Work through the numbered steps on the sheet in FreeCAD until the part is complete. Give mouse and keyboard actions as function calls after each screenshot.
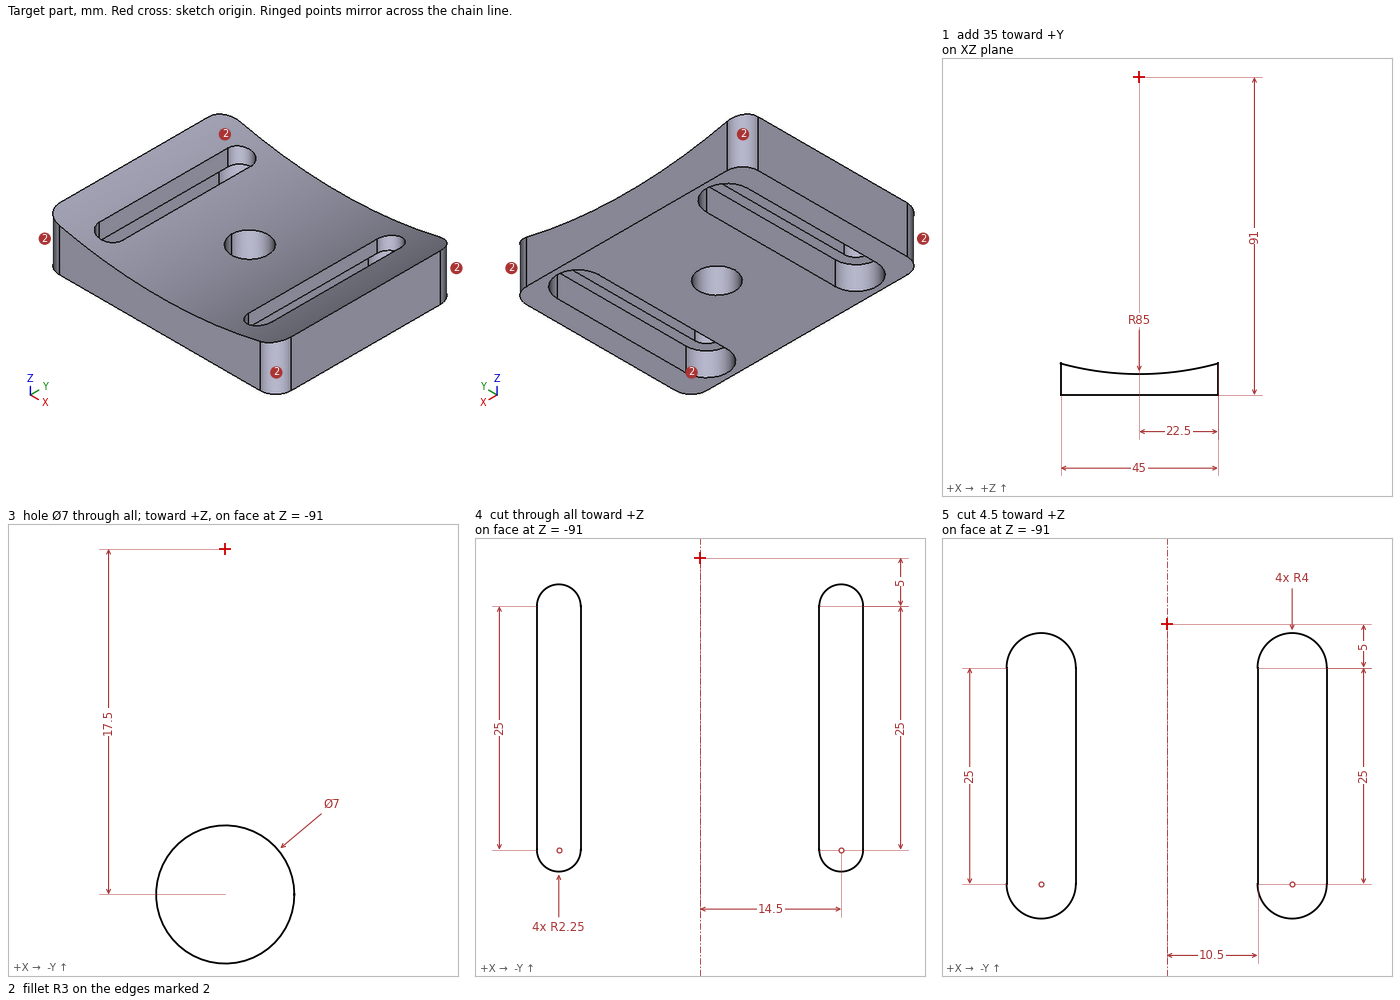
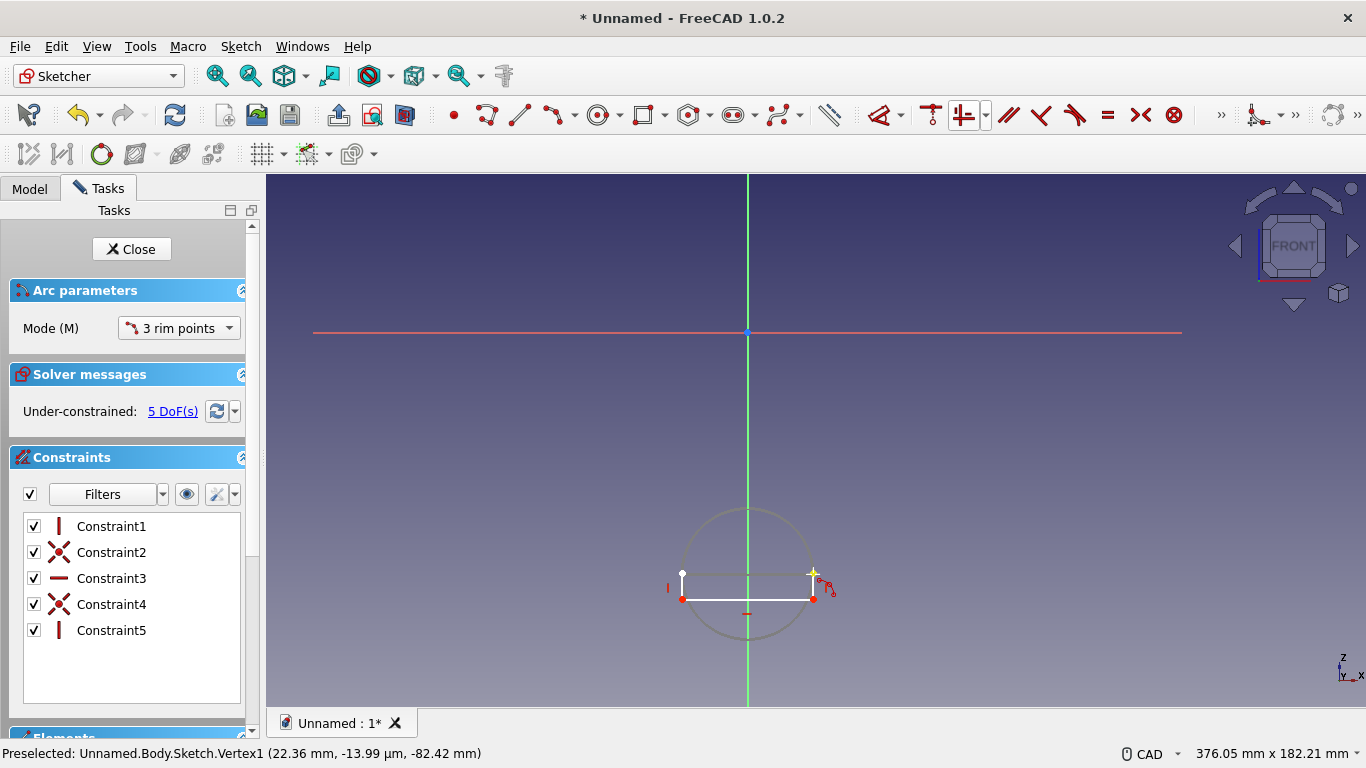
scroll(734, 581, up, 4)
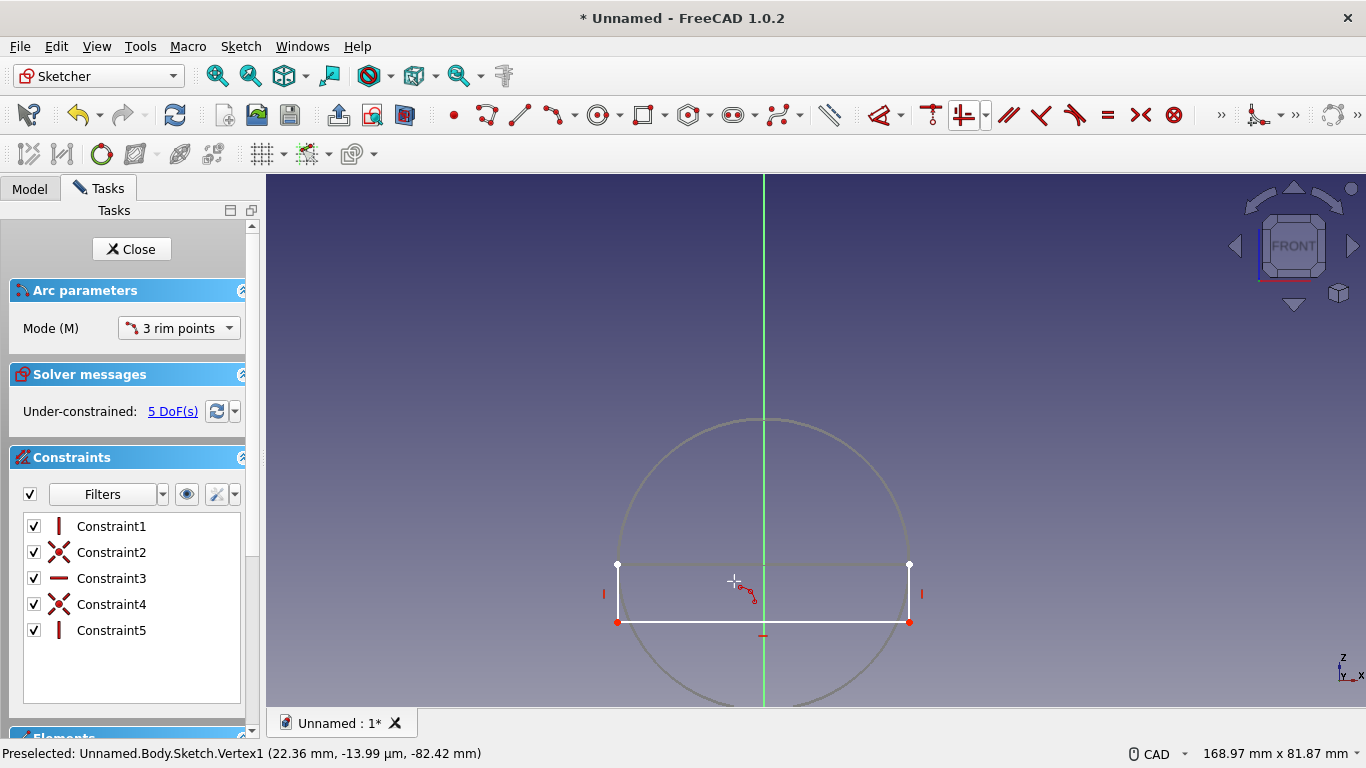
click(734, 581)
key(Escape)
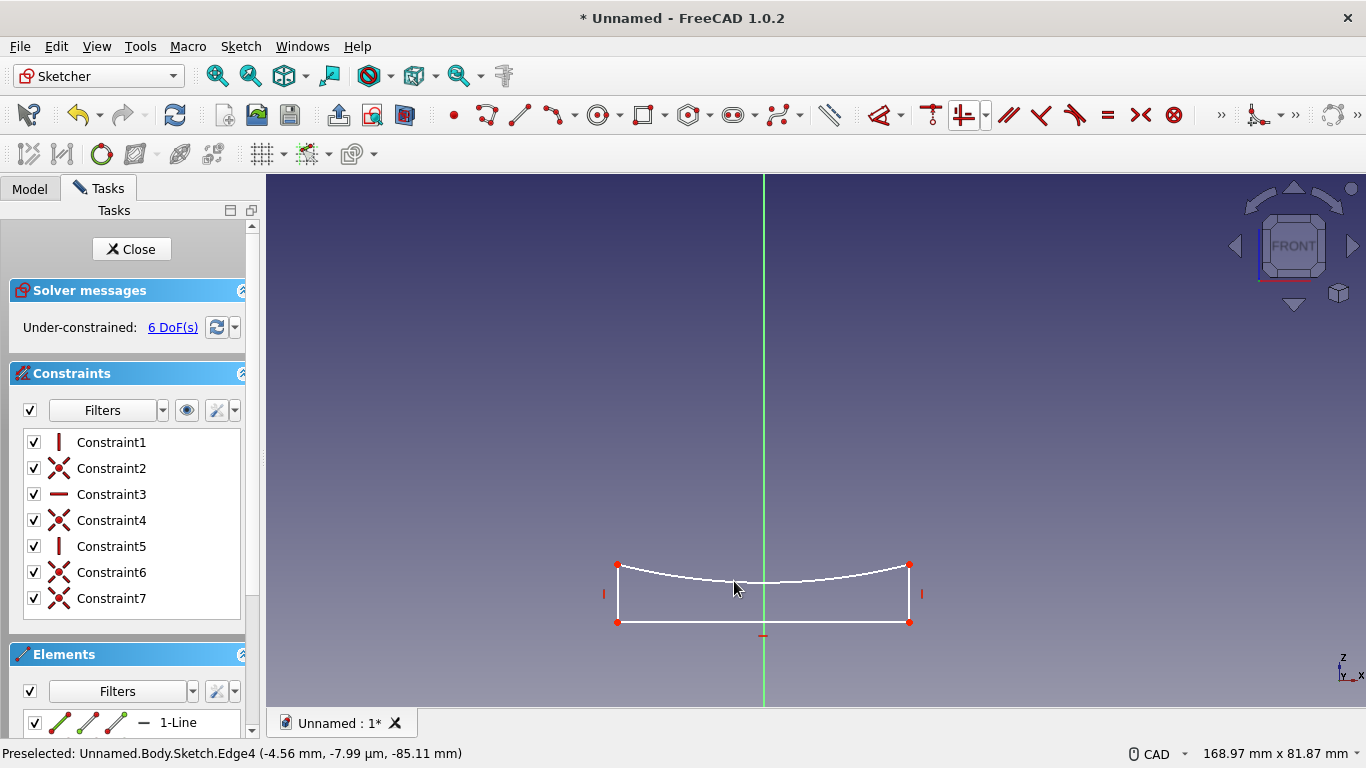
scroll(728, 582, down, 3)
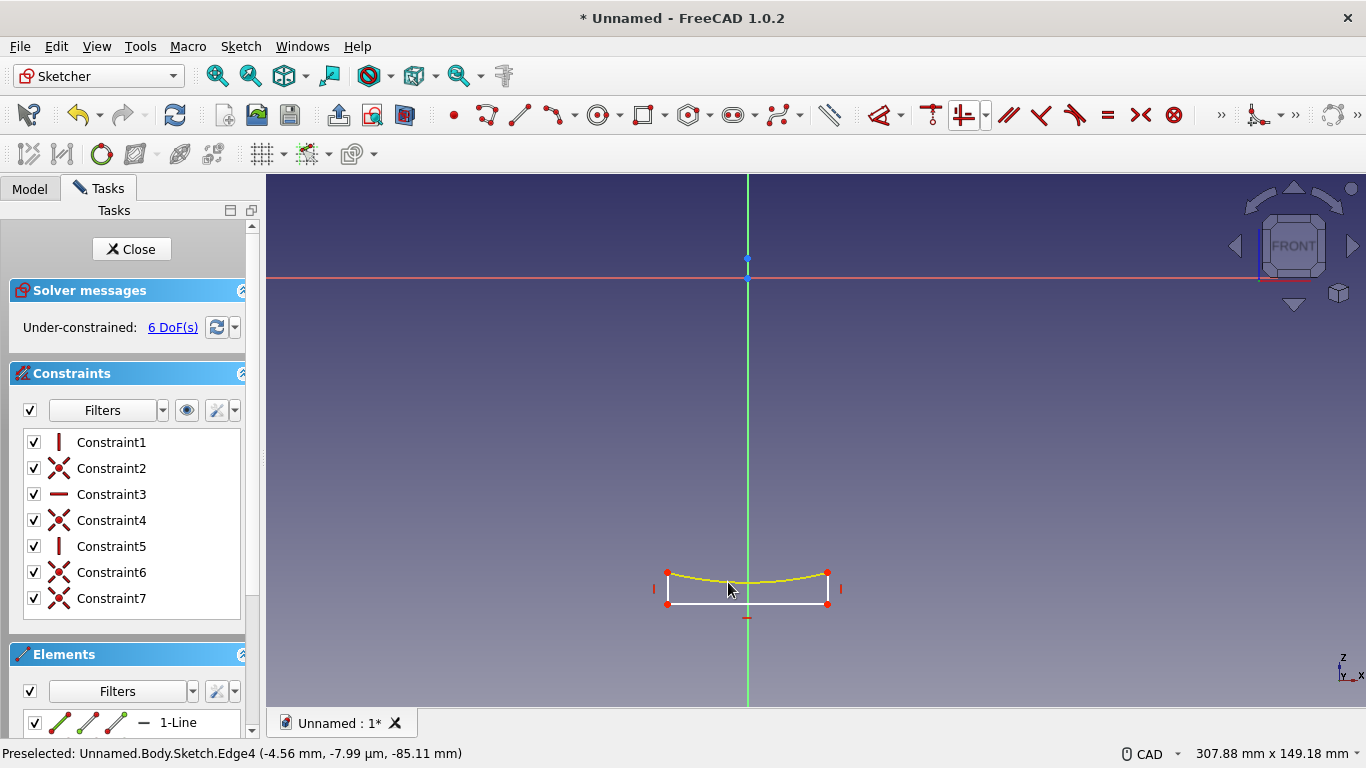
drag(738, 248, 758, 288)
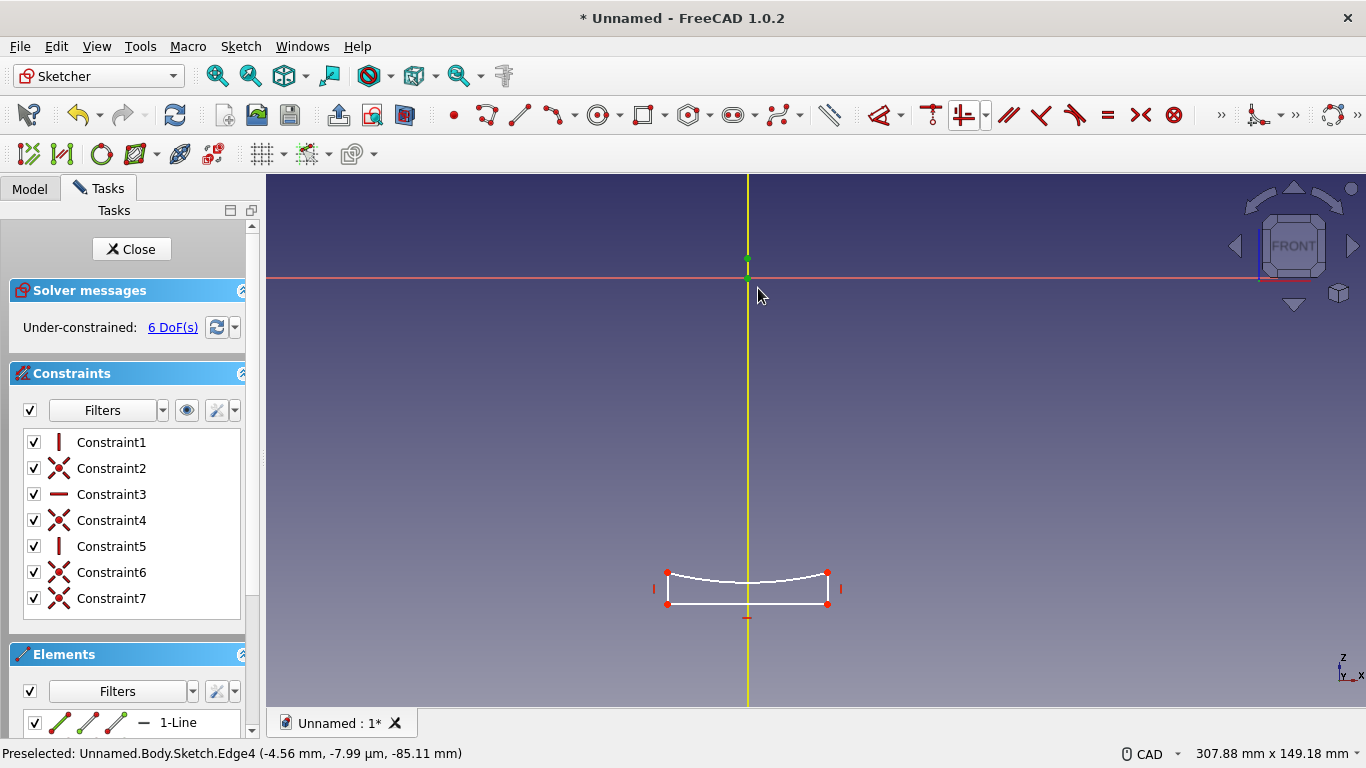
key(c)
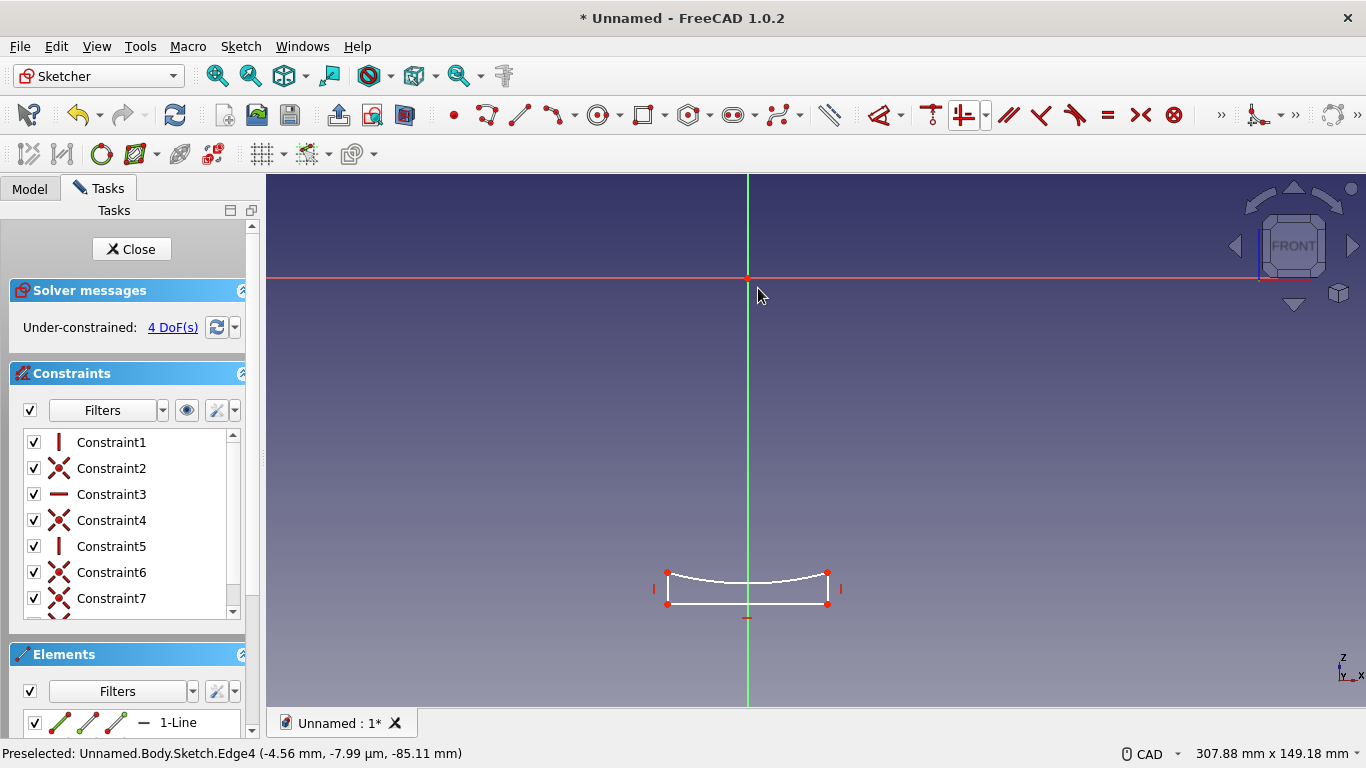
click(878, 116)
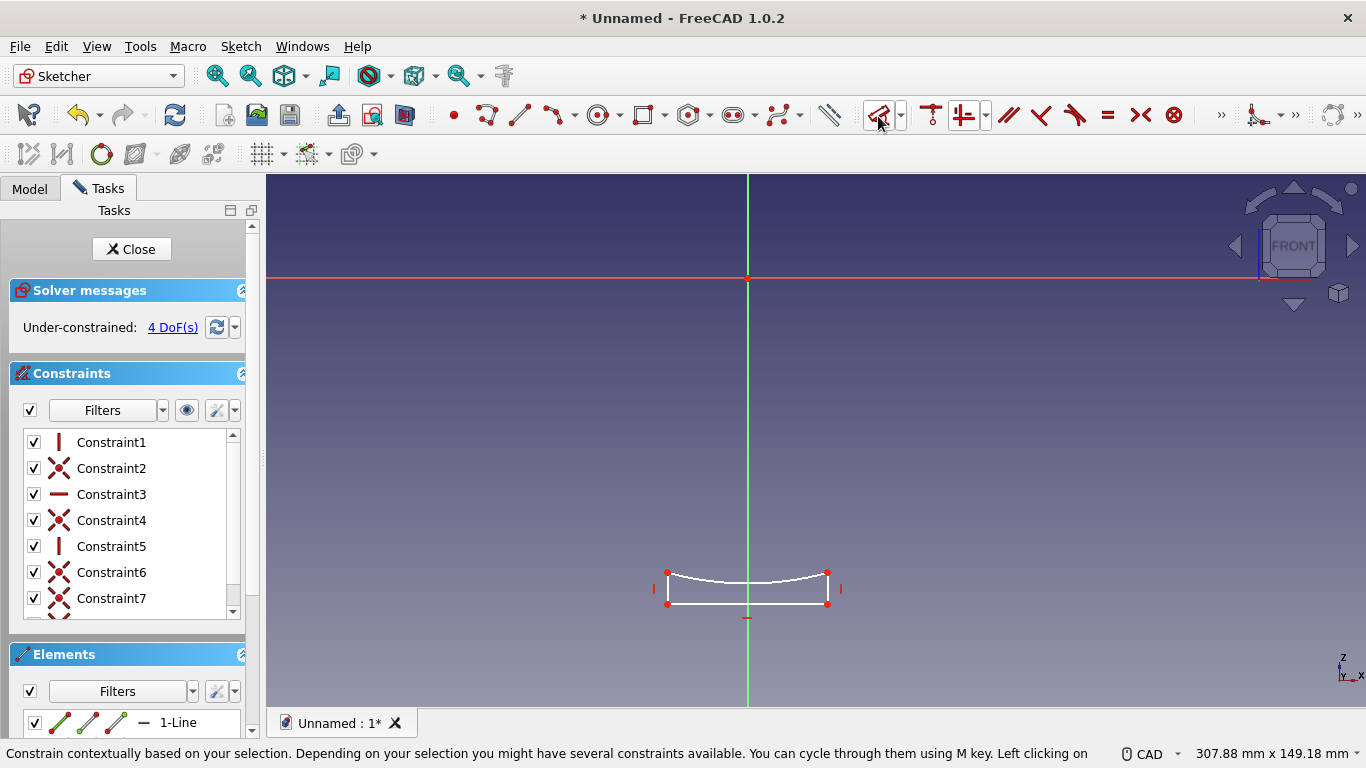
click(715, 582)
click(555, 555)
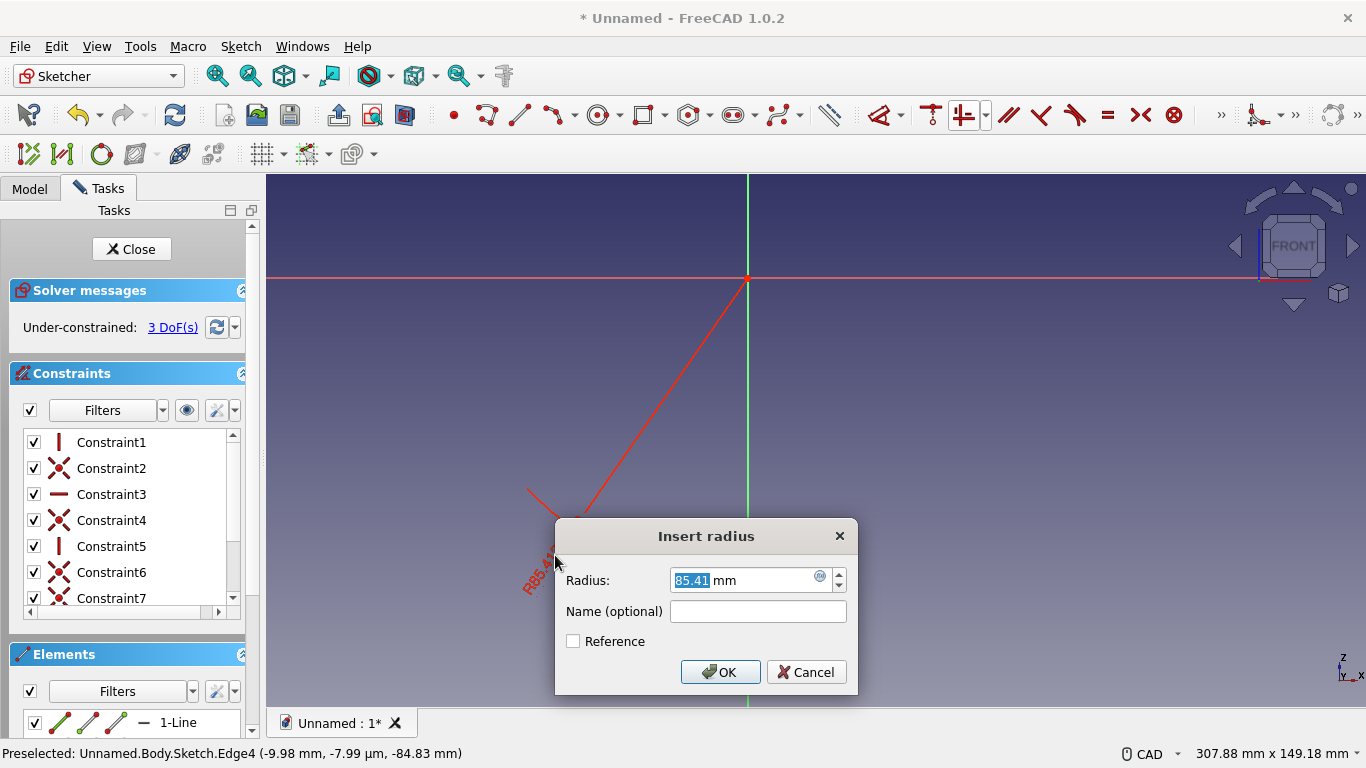
text(85)
key(Return)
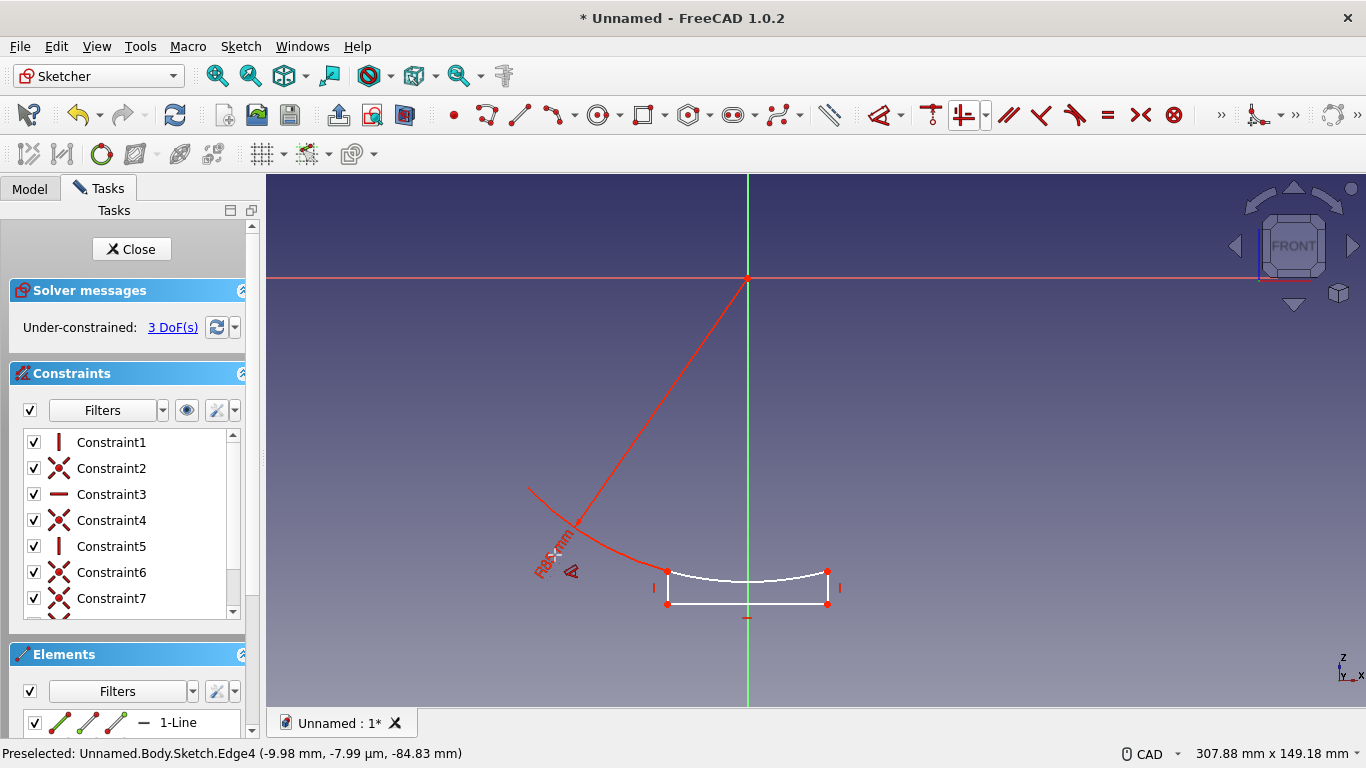
click(780, 604)
click(711, 638)